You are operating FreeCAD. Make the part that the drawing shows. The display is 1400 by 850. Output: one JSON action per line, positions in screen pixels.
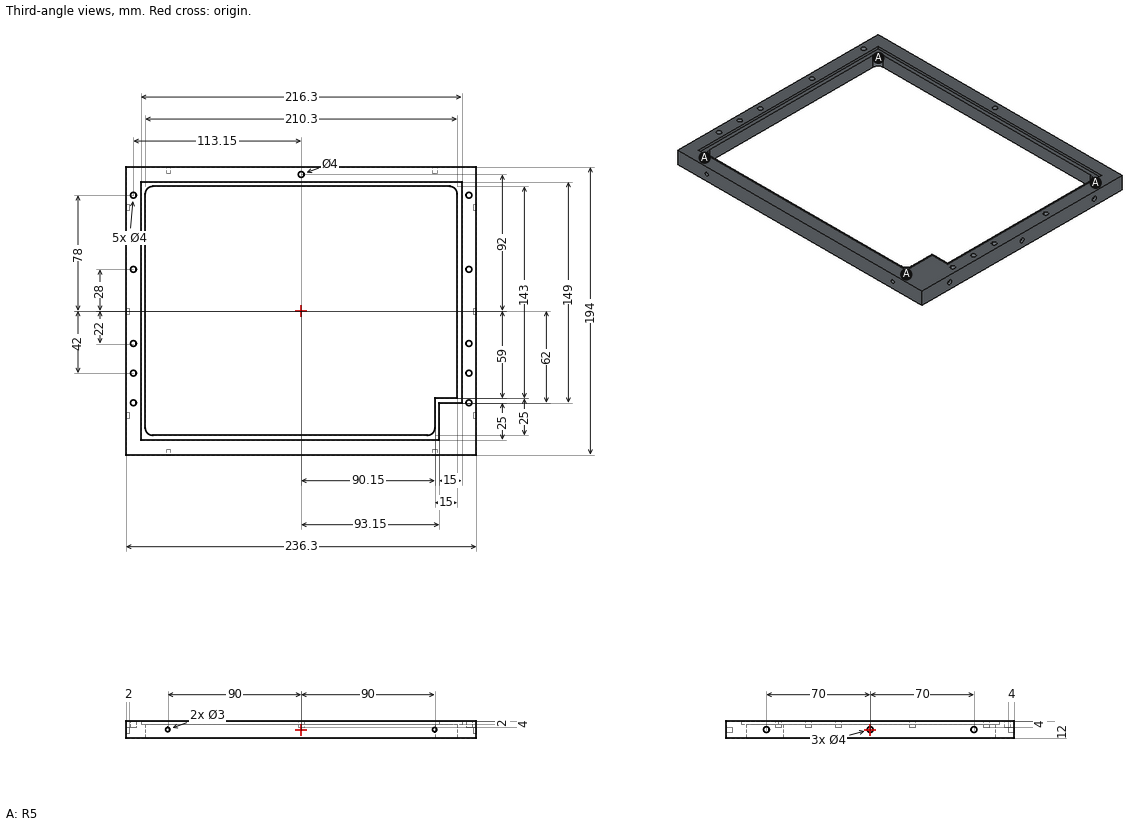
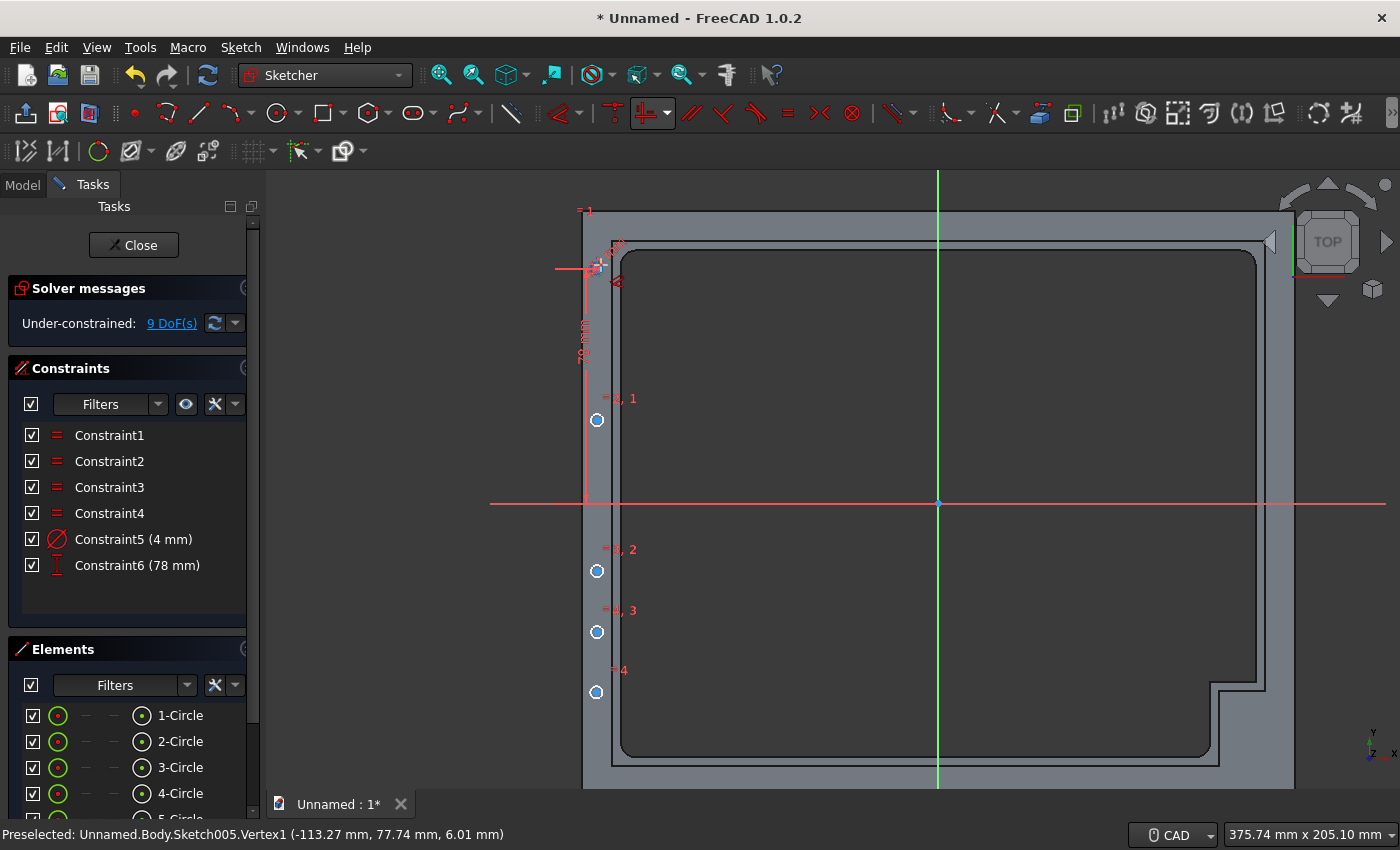
{"action": "left_click", "coordinate": [597, 420]}
{"action": "left_click", "coordinate": [972, 462]}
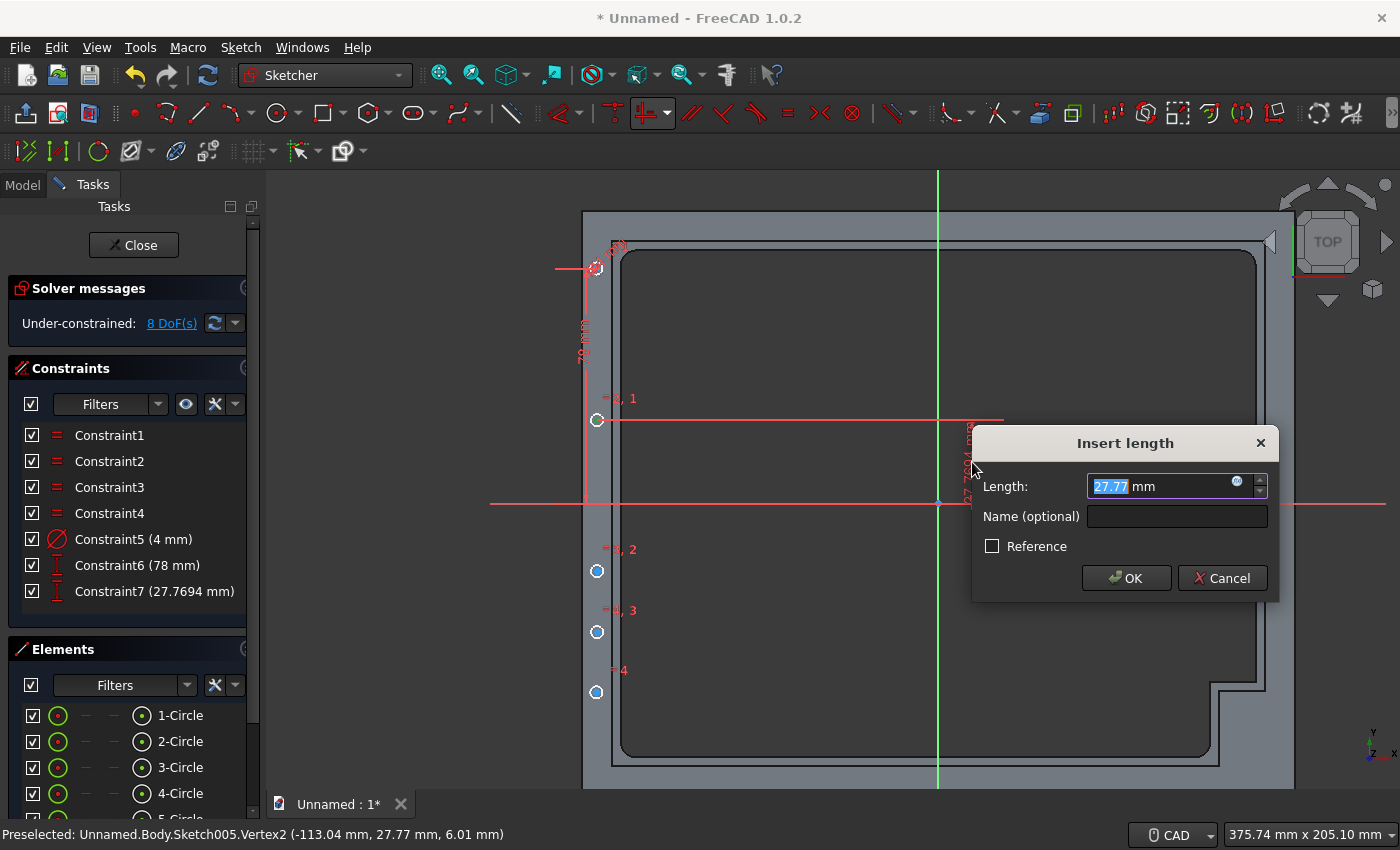
{"action": "type", "text": "28"}
{"action": "key", "text": "Return"}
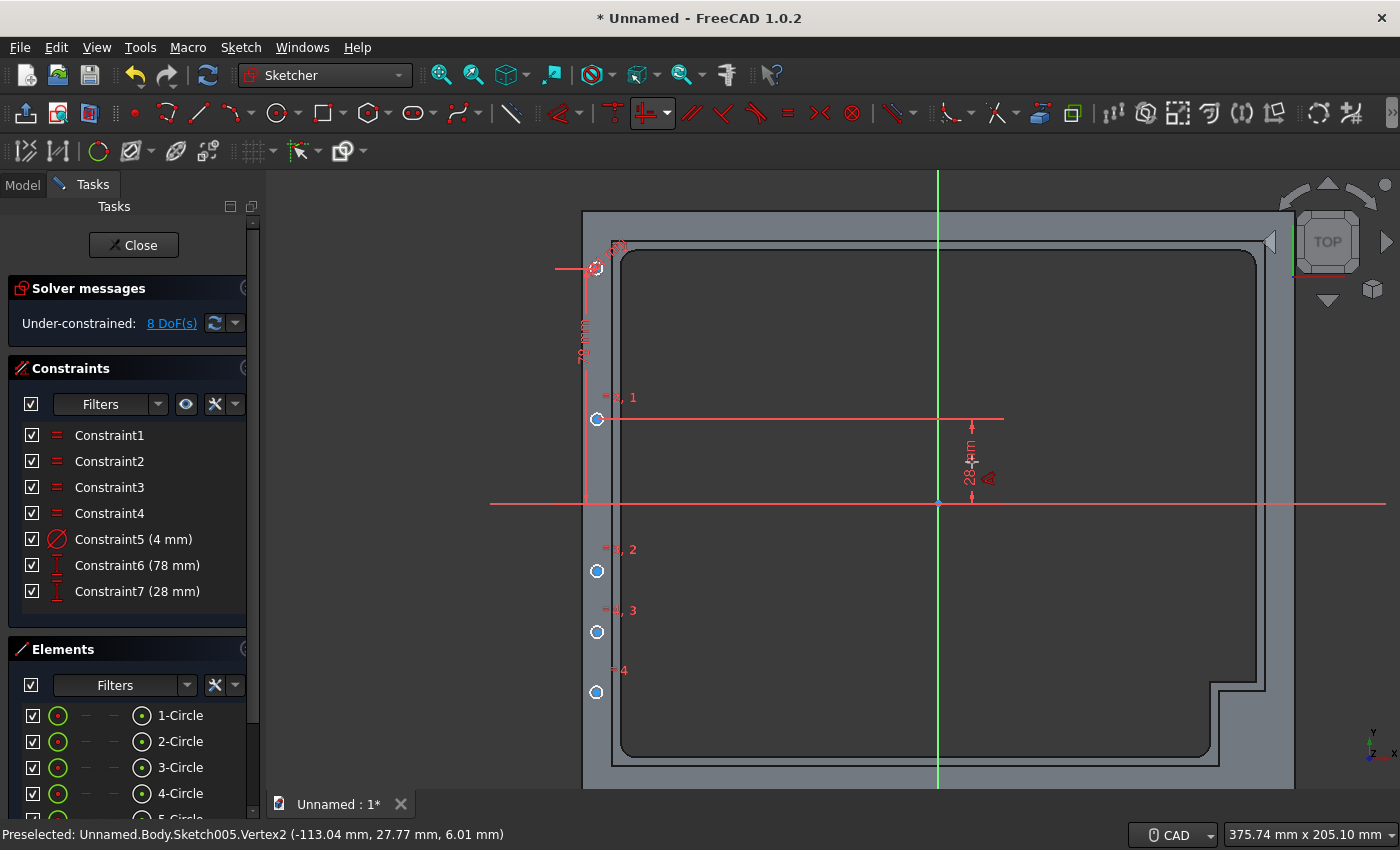
{"action": "left_click", "coordinate": [597, 571]}
{"action": "left_click", "coordinate": [972, 538]}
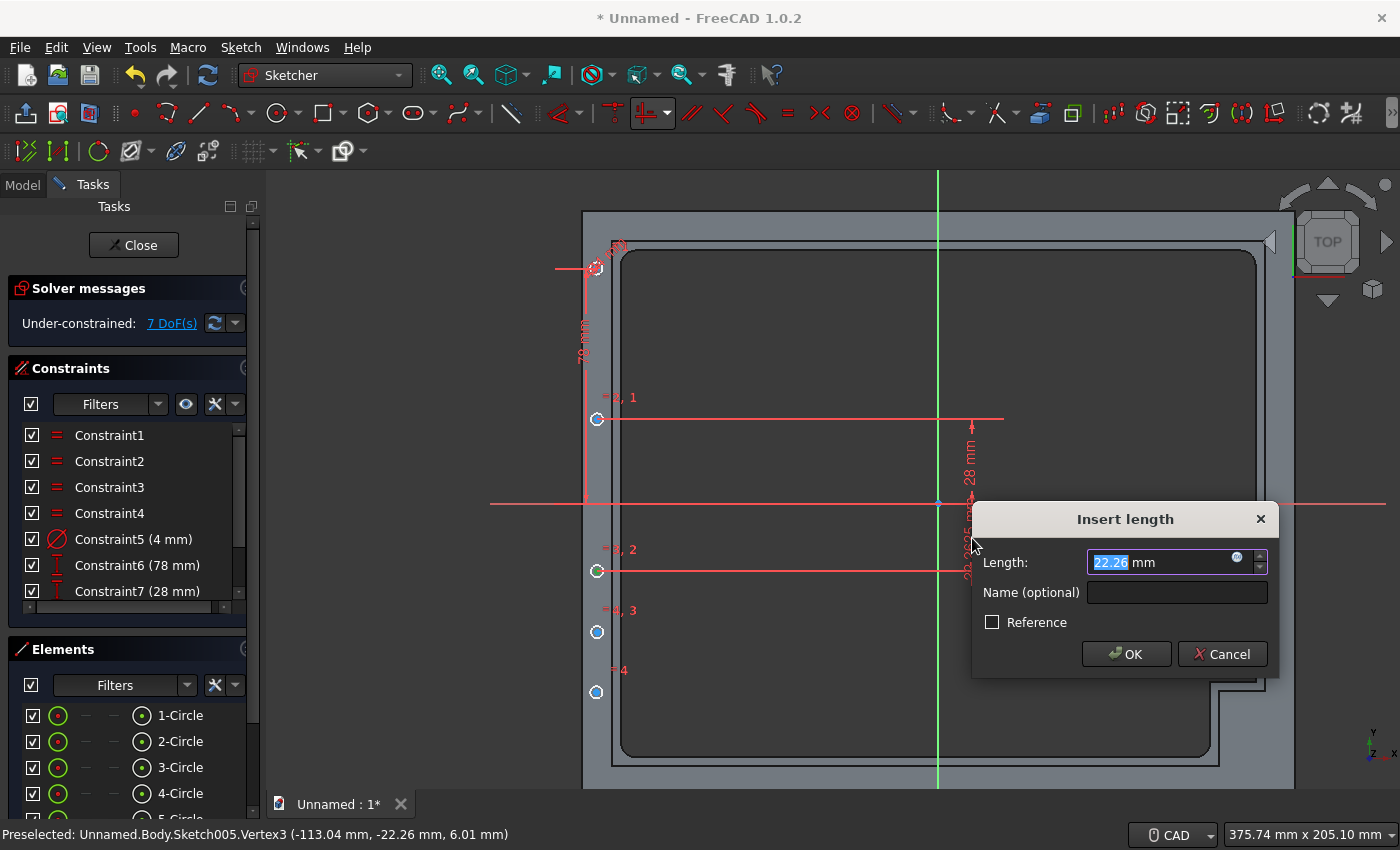
{"action": "type", "text": "22"}
{"action": "key", "text": "Return"}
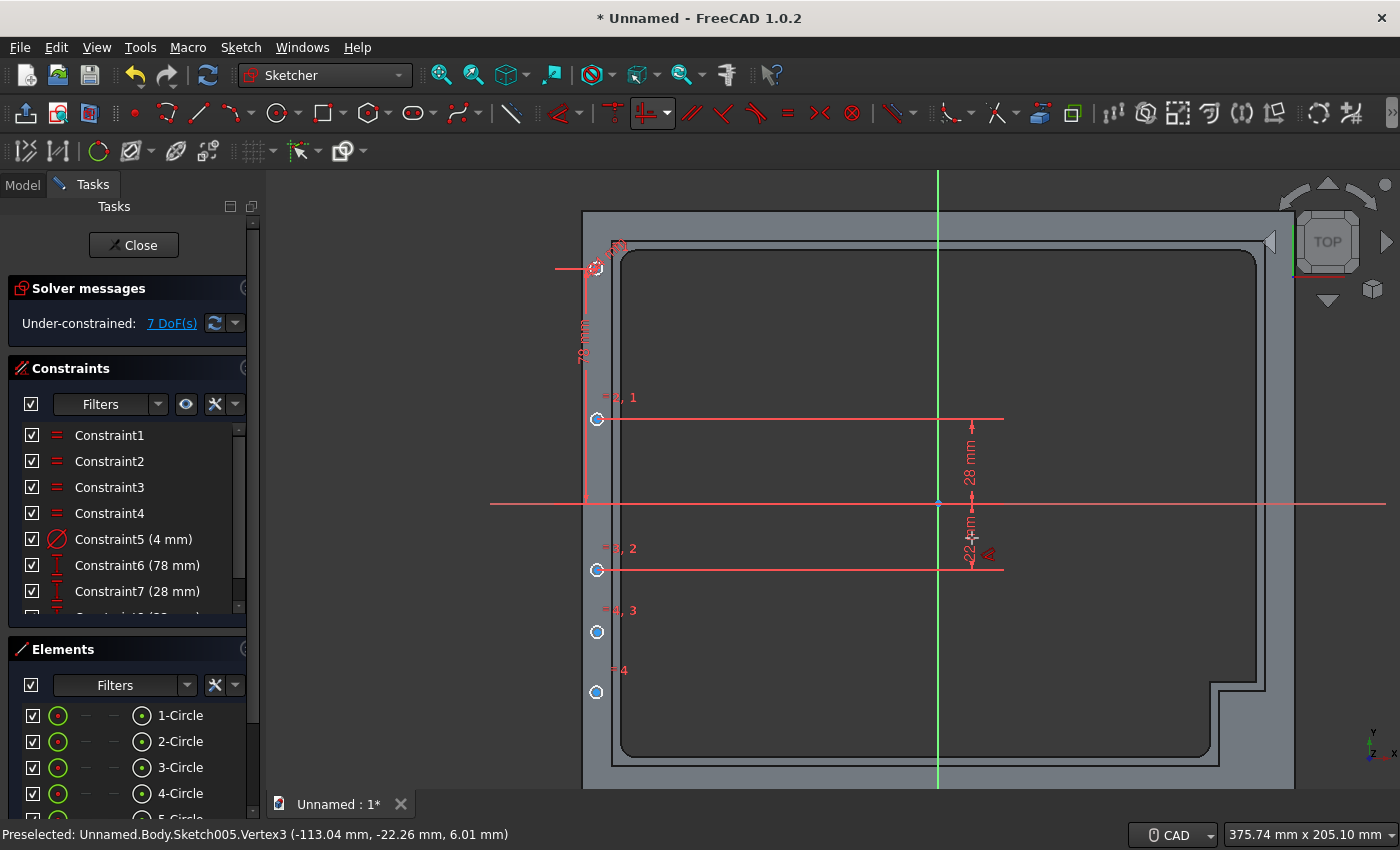
{"action": "left_click", "coordinate": [597, 632]}
{"action": "left_click", "coordinate": [972, 568]}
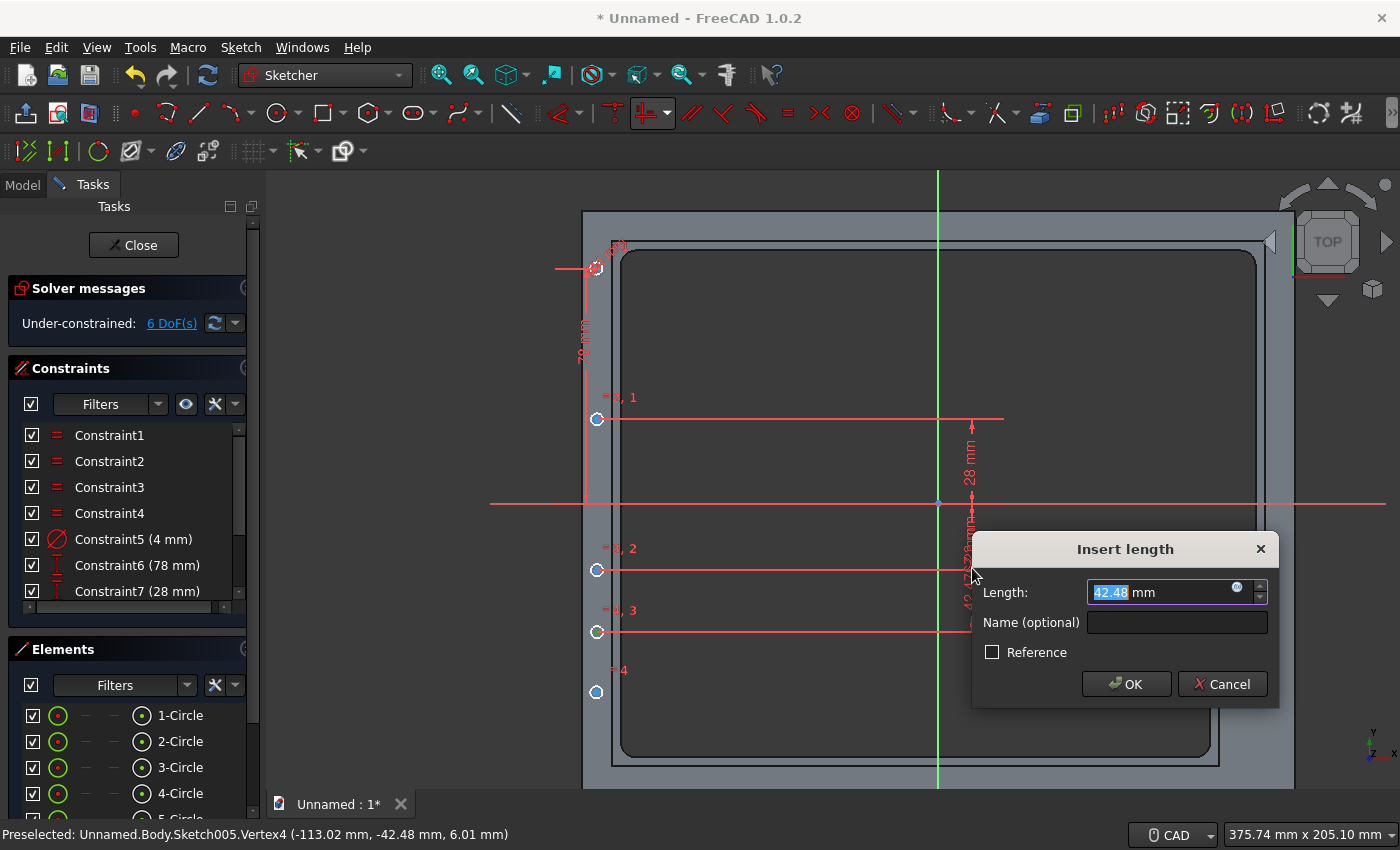
{"action": "type", "text": "42"}
{"action": "key", "text": "Return"}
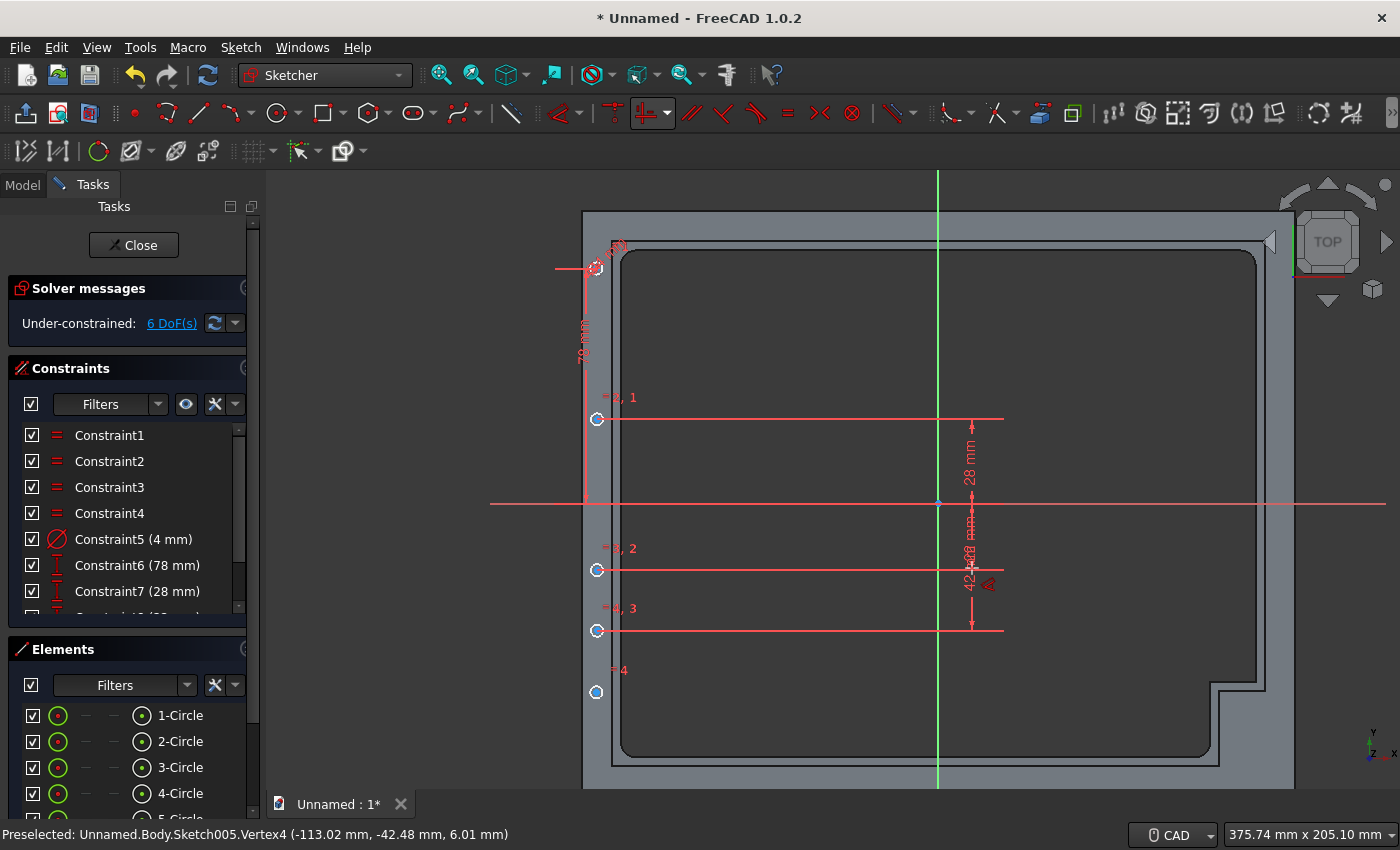
{"action": "left_click", "coordinate": [596, 692]}
{"action": "left_click", "coordinate": [972, 598]}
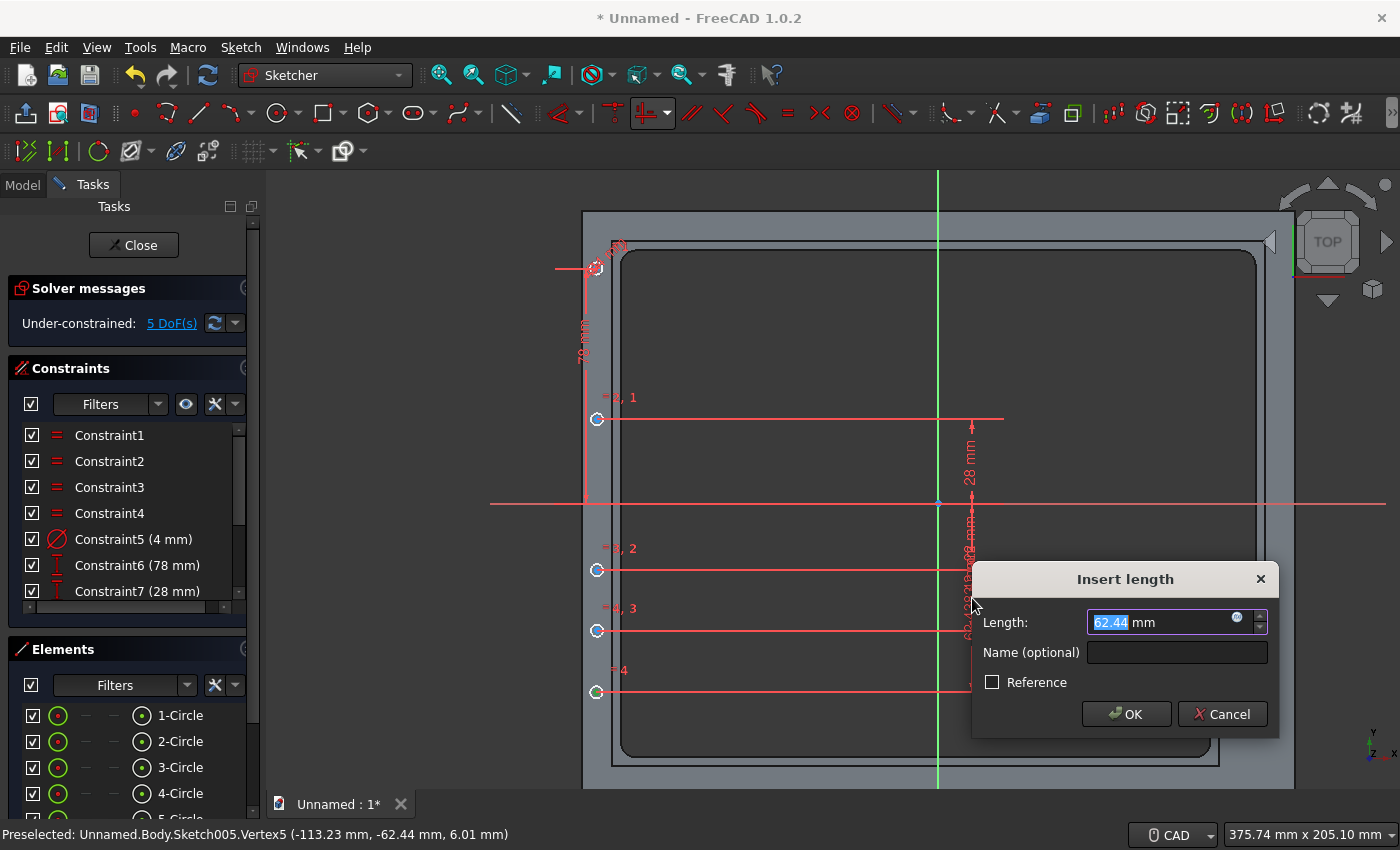
{"action": "type", "text": "62"}
{"action": "key", "text": "Return"}